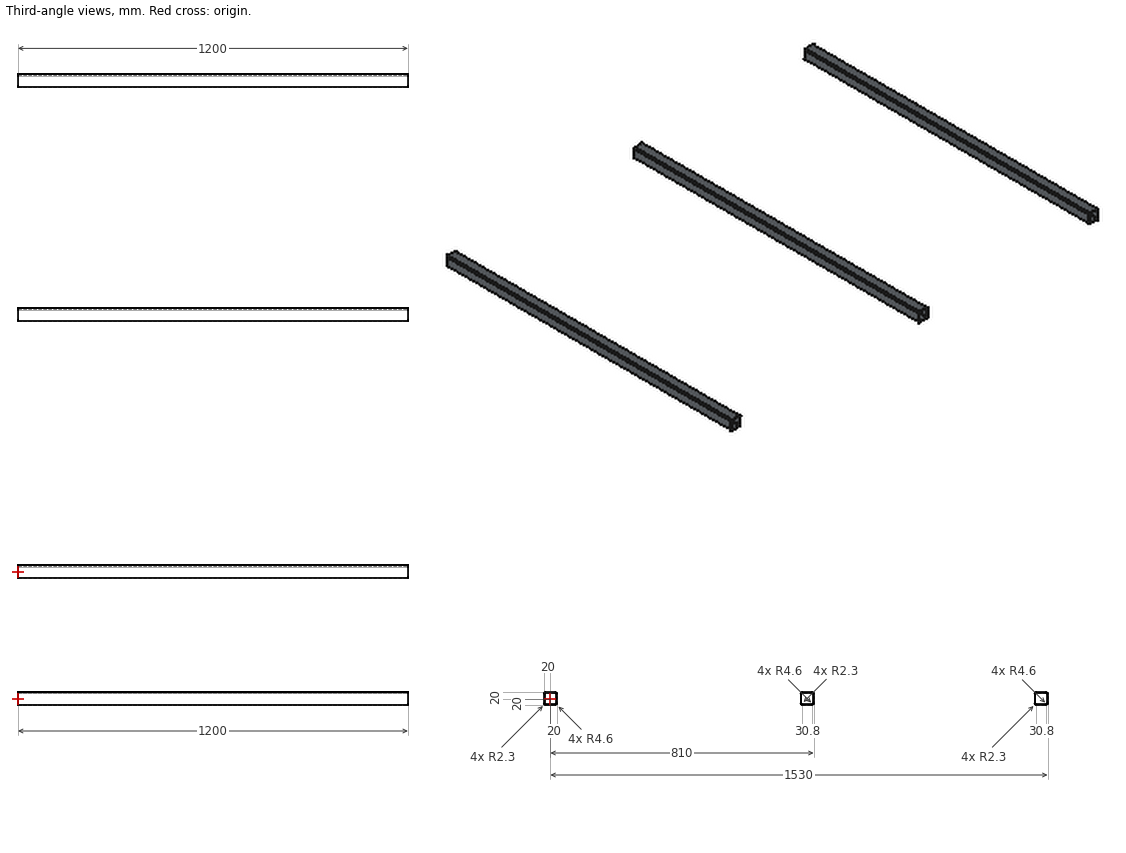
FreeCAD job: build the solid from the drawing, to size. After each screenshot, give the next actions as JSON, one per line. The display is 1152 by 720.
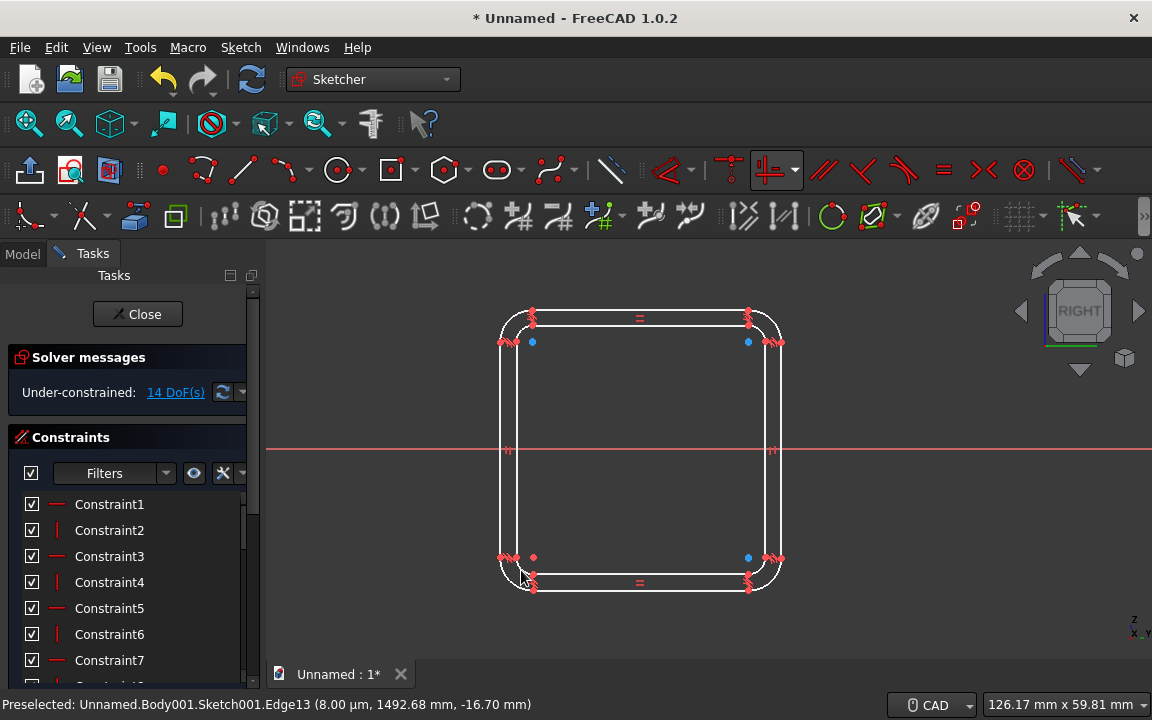
{"action": "left_click", "coordinate": [518, 314]}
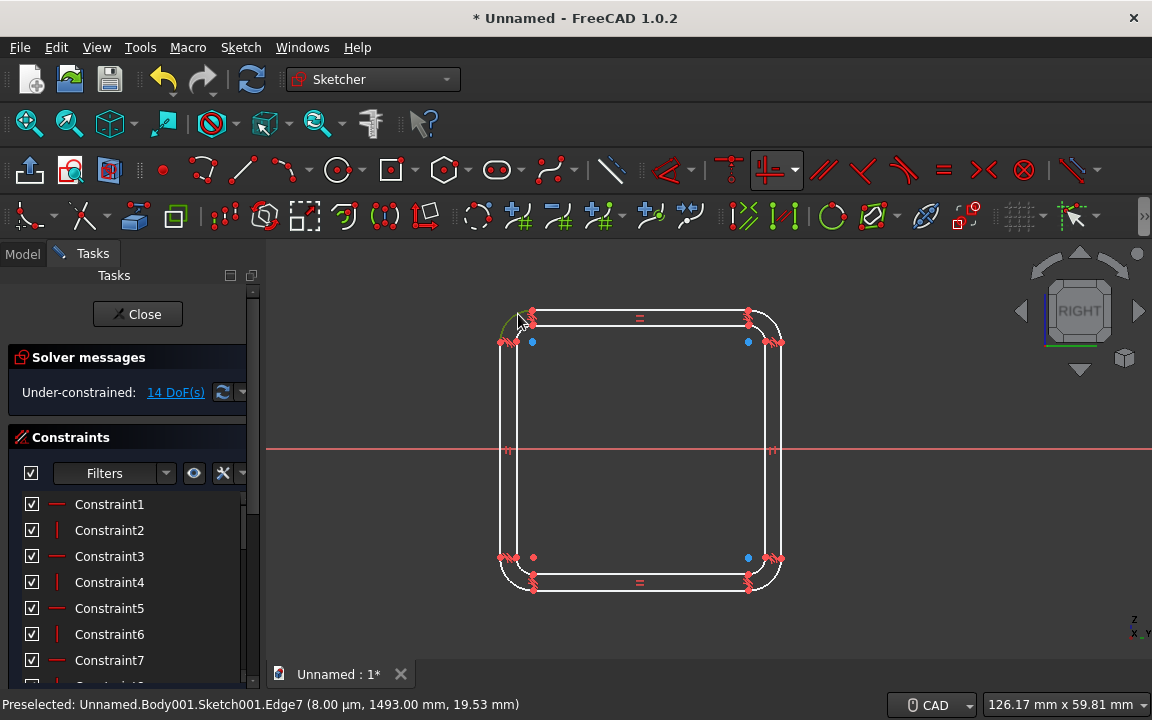
{"action": "left_click", "coordinate": [521, 330]}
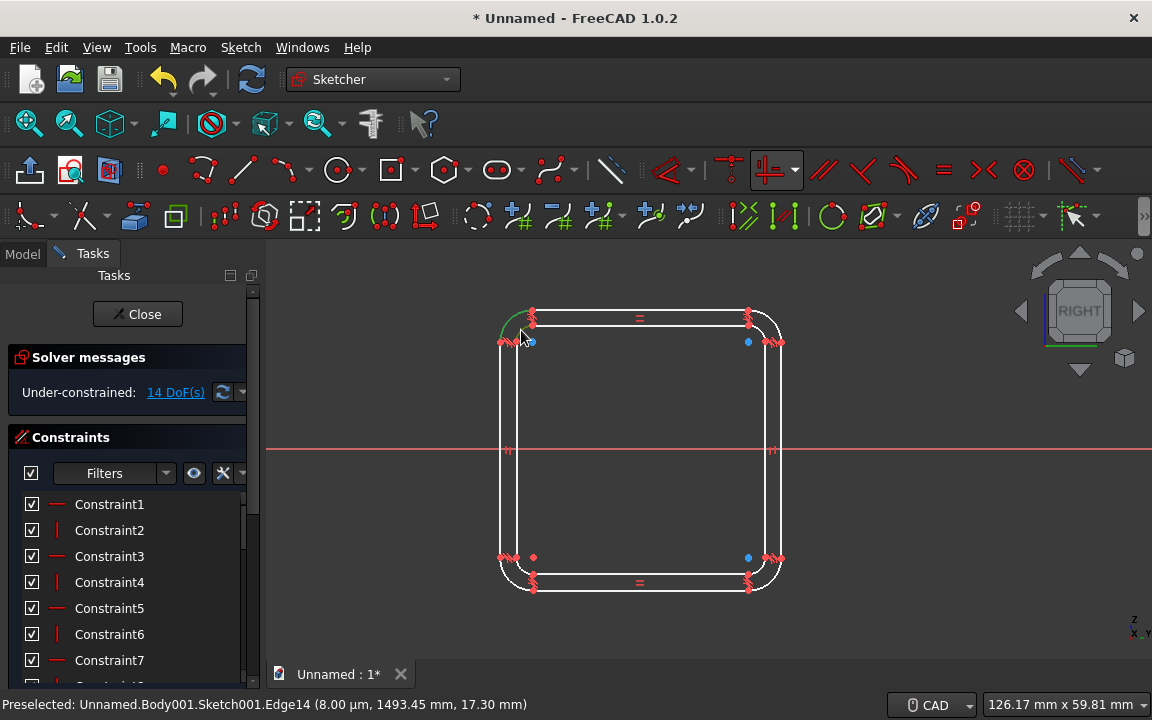
{"action": "left_click", "coordinate": [730, 170]}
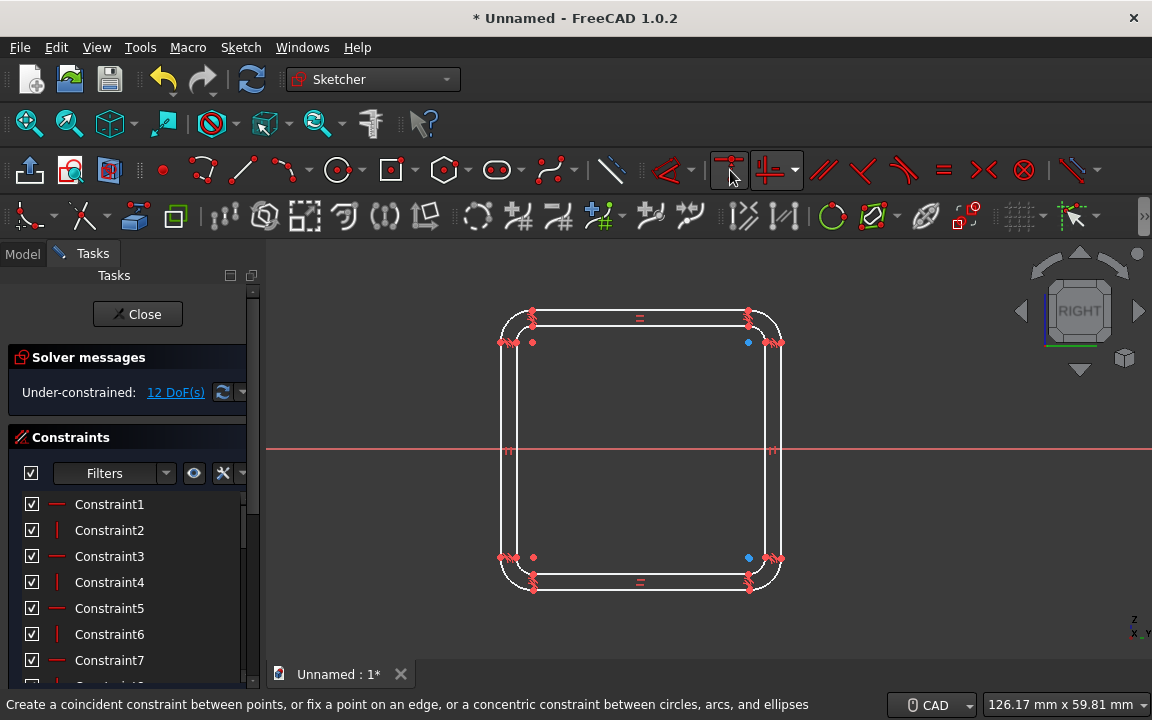
{"action": "left_click", "coordinate": [778, 328]}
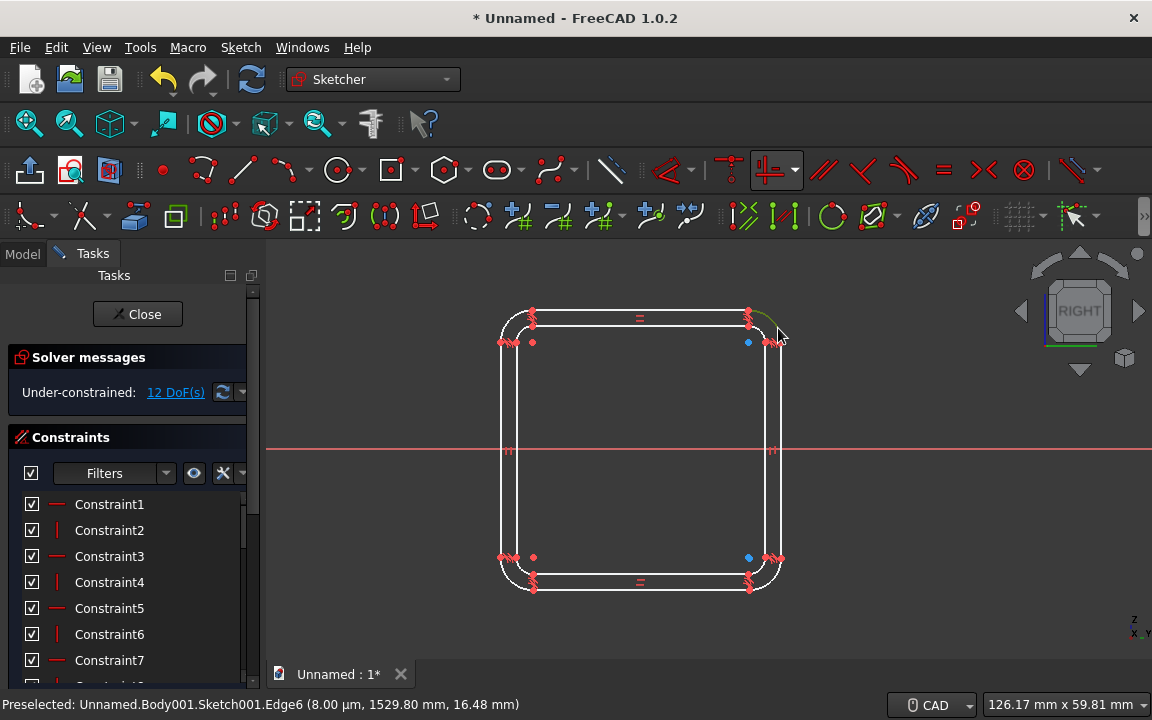
{"action": "left_click", "coordinate": [760, 331]}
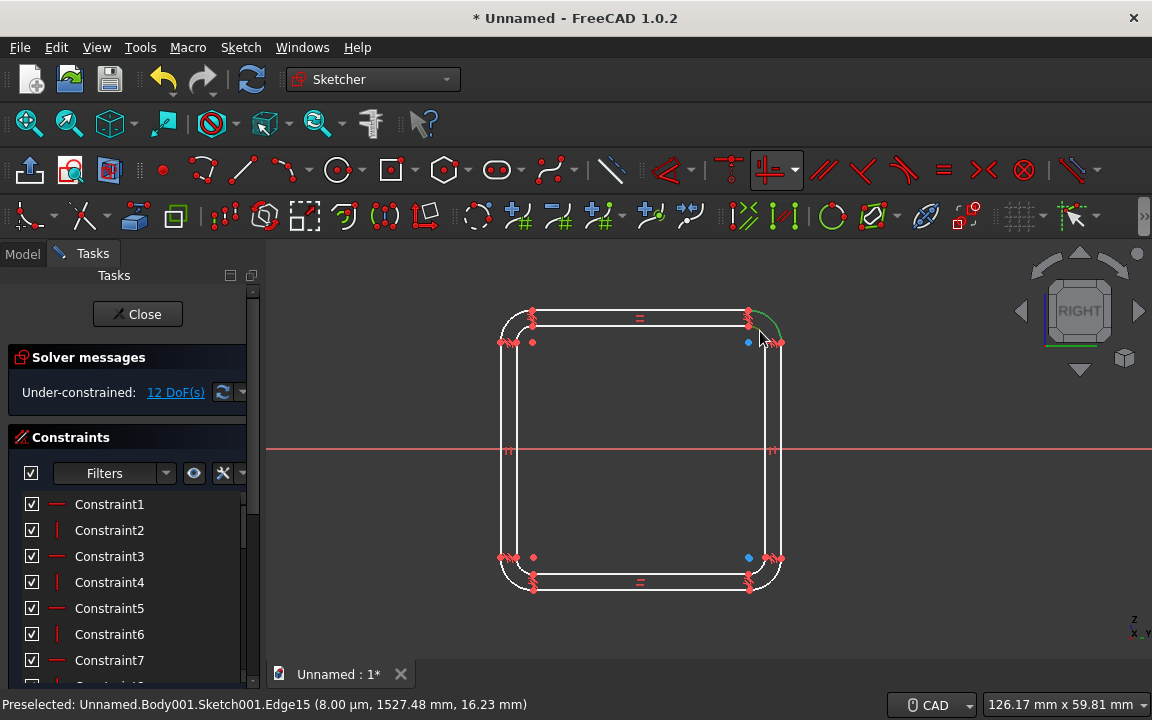
{"action": "key", "text": "c"}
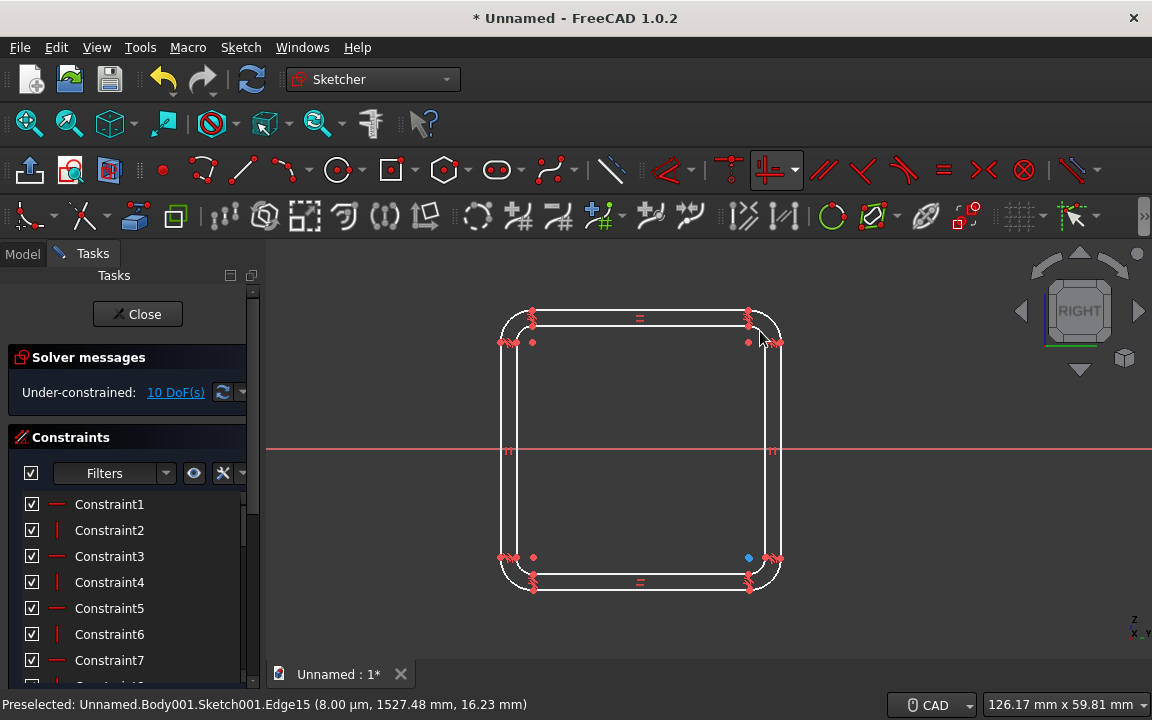
{"action": "left_click", "coordinate": [764, 587]}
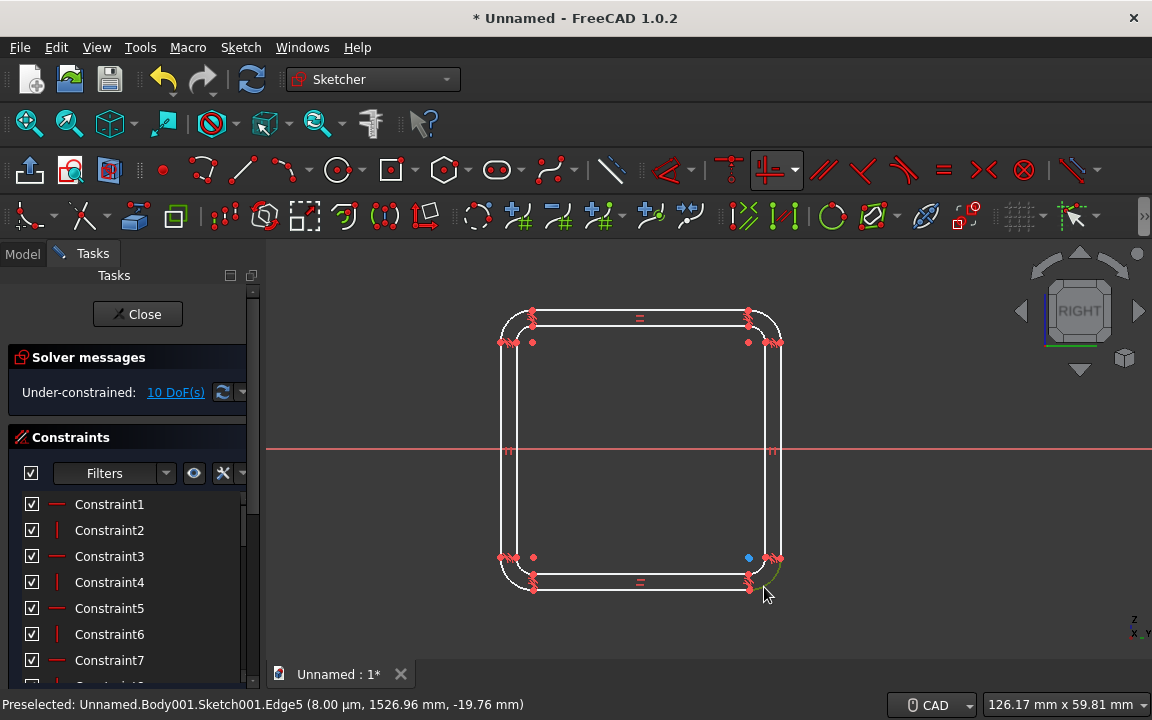
{"action": "left_click", "coordinate": [777, 328]}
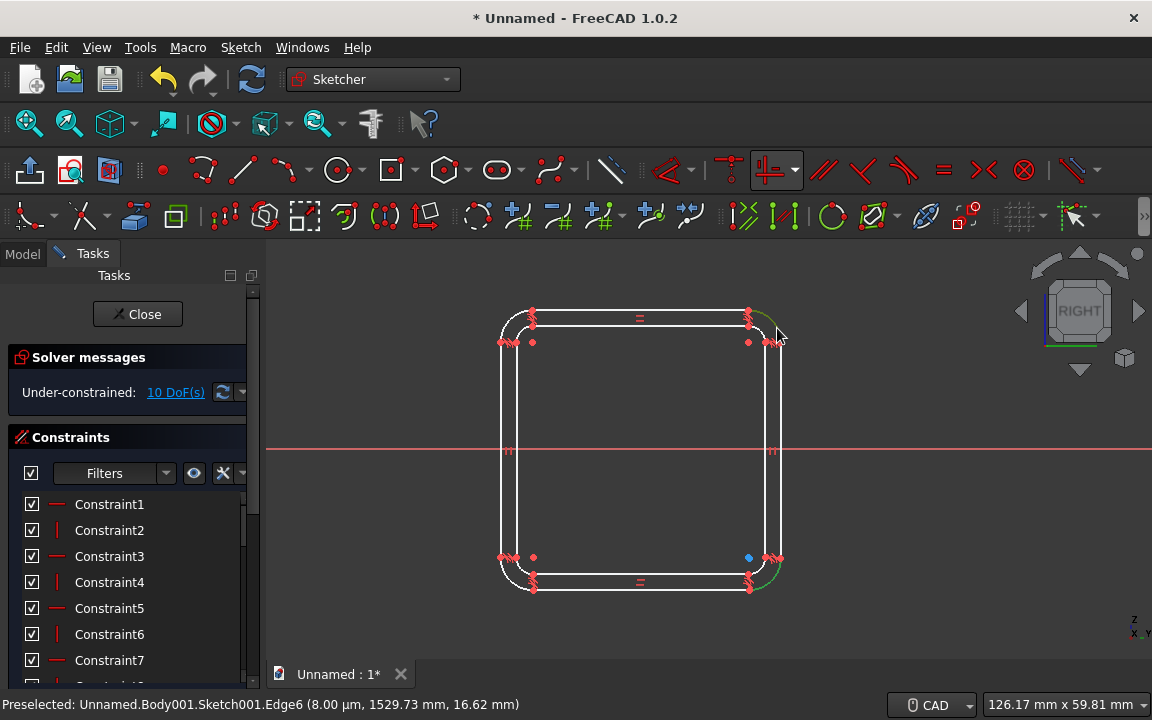
{"action": "left_click", "coordinate": [518, 314]}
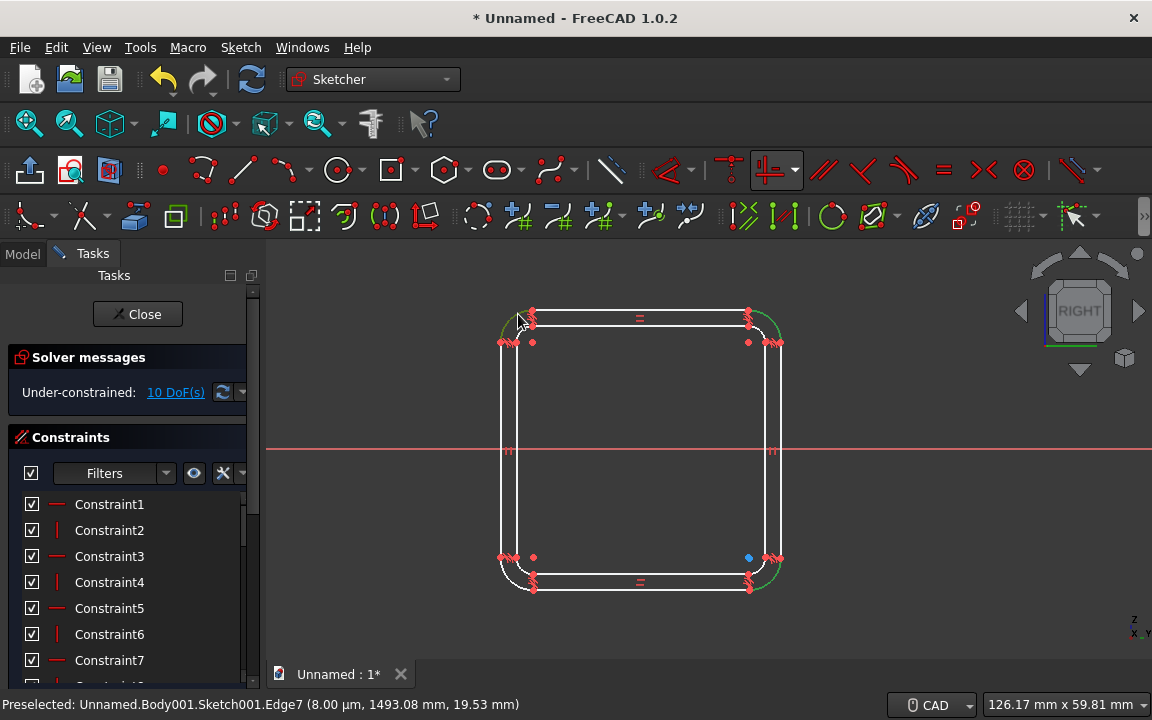
{"action": "left_click", "coordinate": [504, 572]}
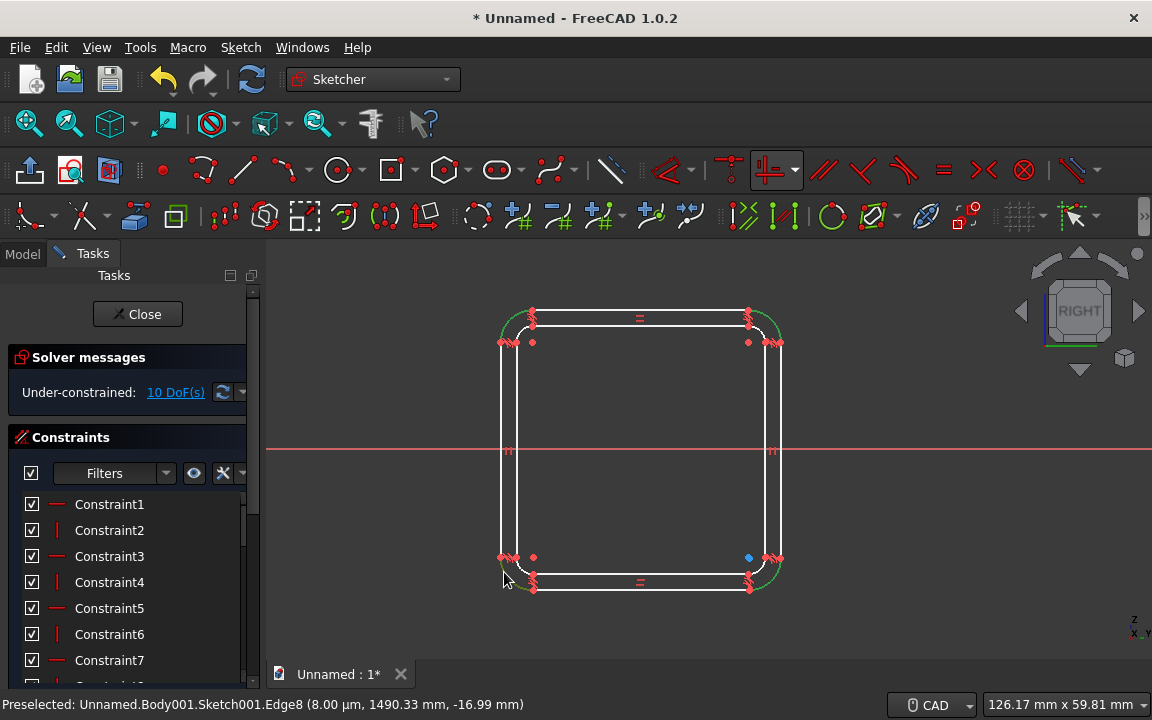
{"action": "key", "text": "e"}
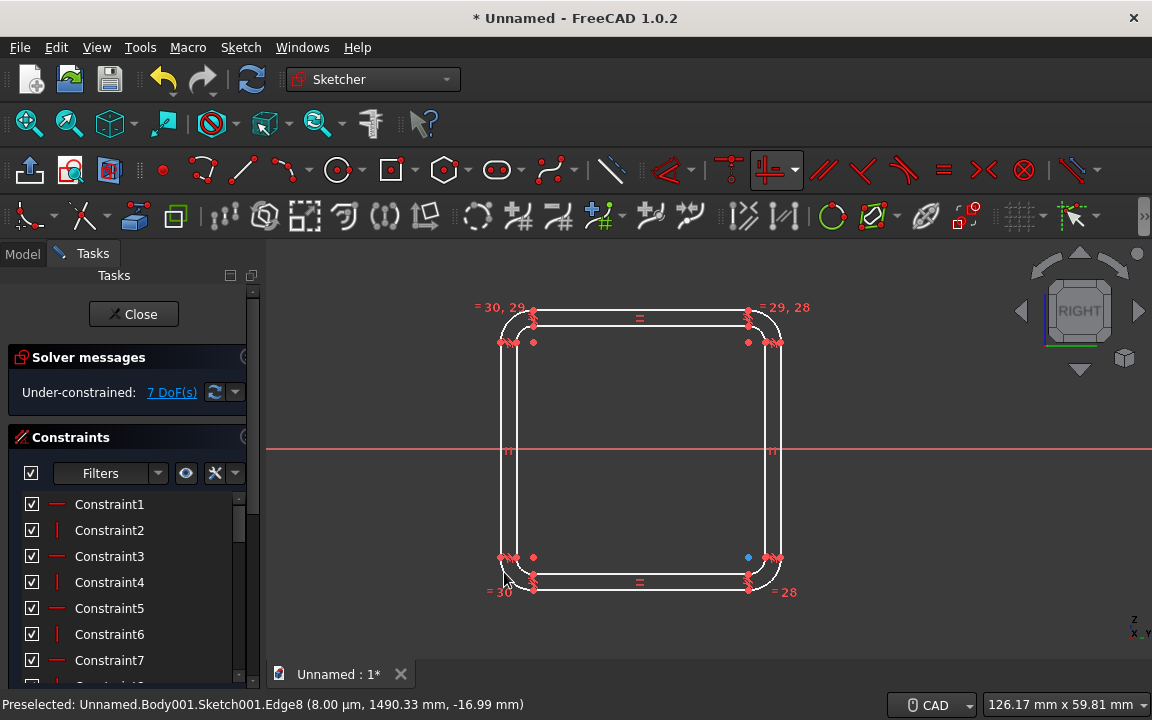
{"action": "left_click", "coordinate": [521, 569]}